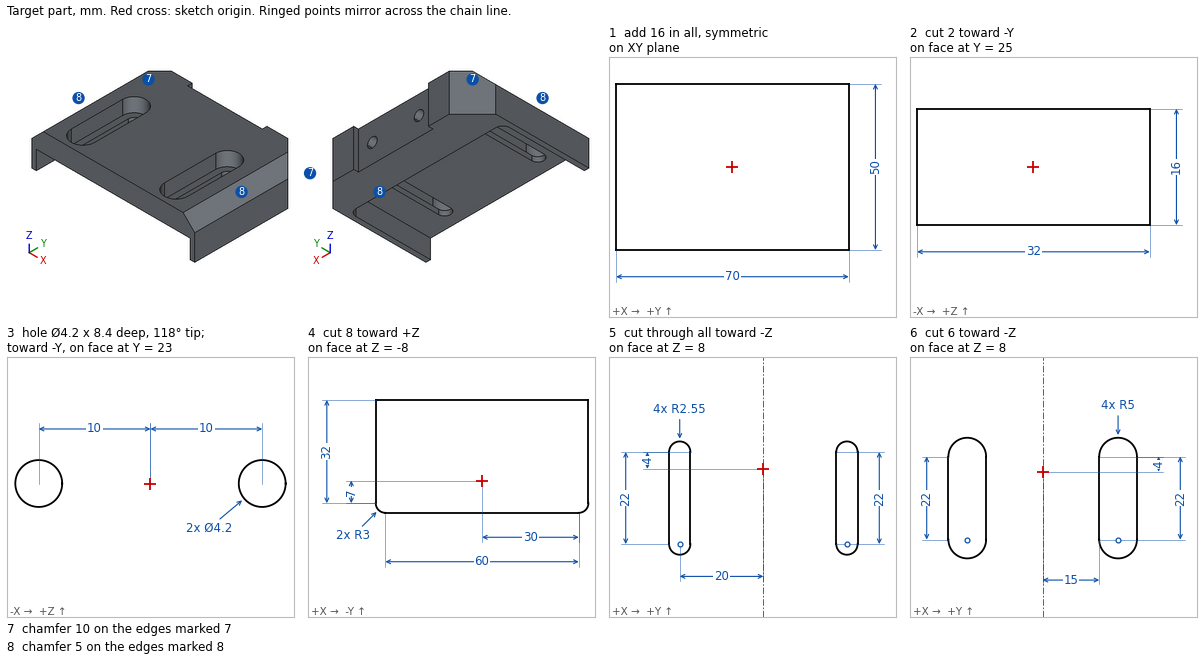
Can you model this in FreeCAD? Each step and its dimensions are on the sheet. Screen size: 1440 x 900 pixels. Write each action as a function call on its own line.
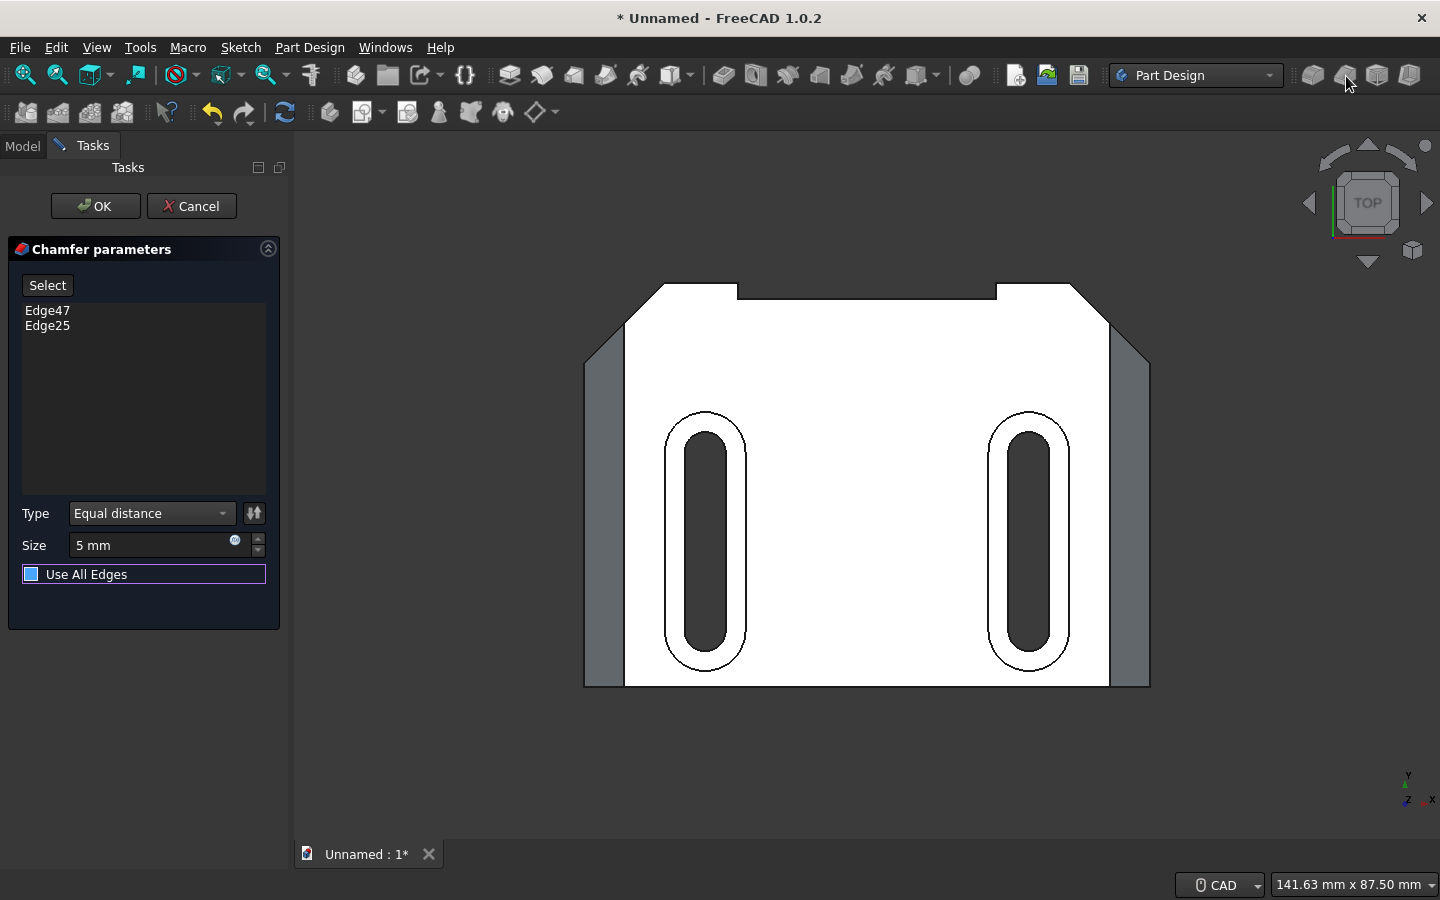
click(96, 206)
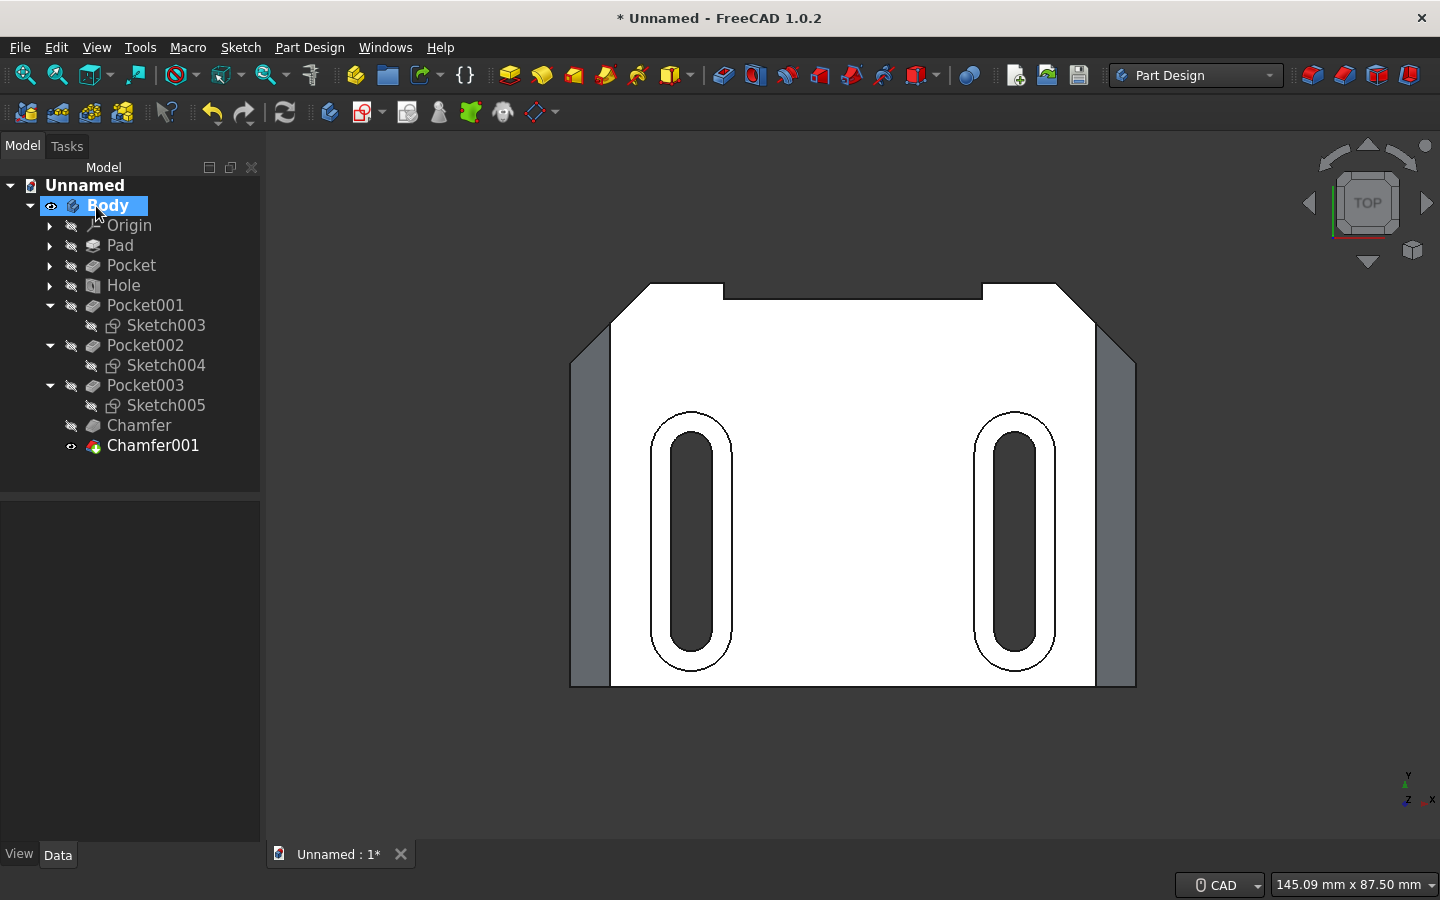
key(0)